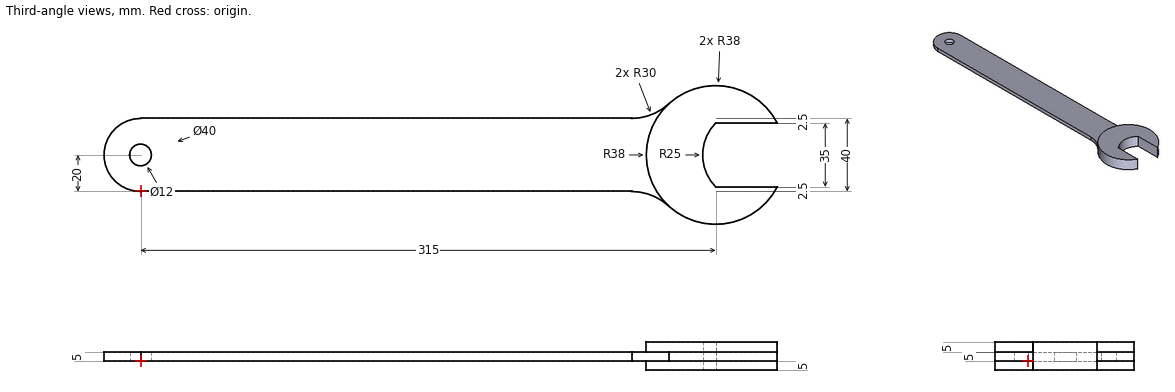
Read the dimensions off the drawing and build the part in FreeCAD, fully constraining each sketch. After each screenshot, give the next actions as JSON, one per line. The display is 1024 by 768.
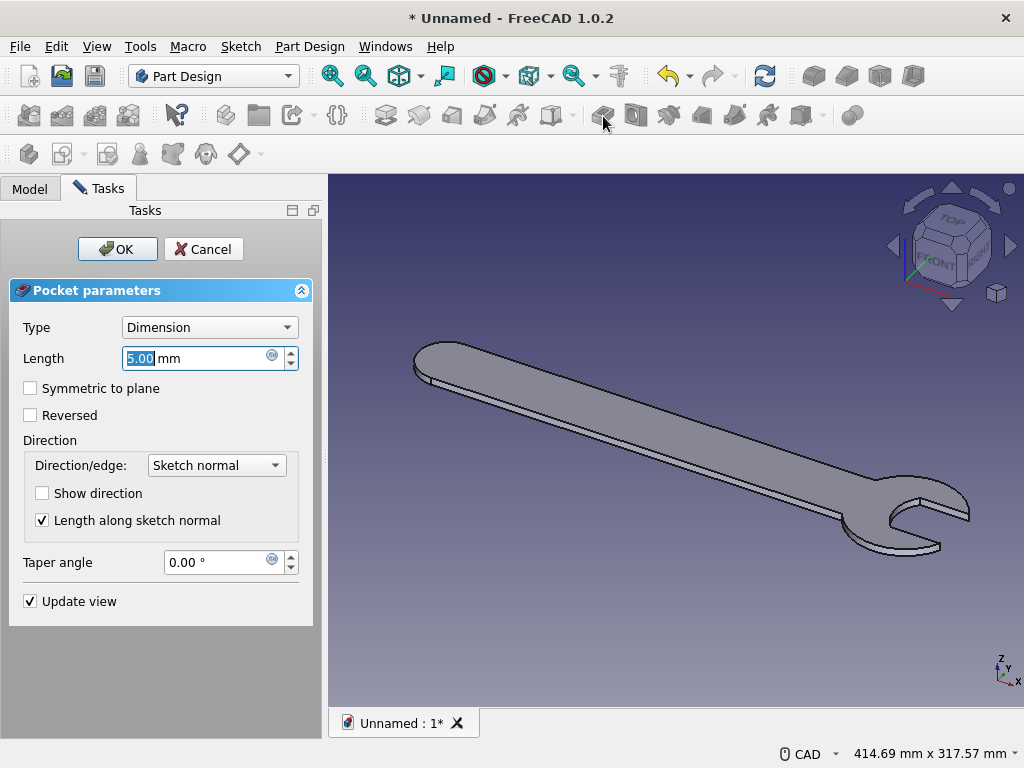
{"action": "type", "text": "5"}
{"action": "key", "text": "Tab"}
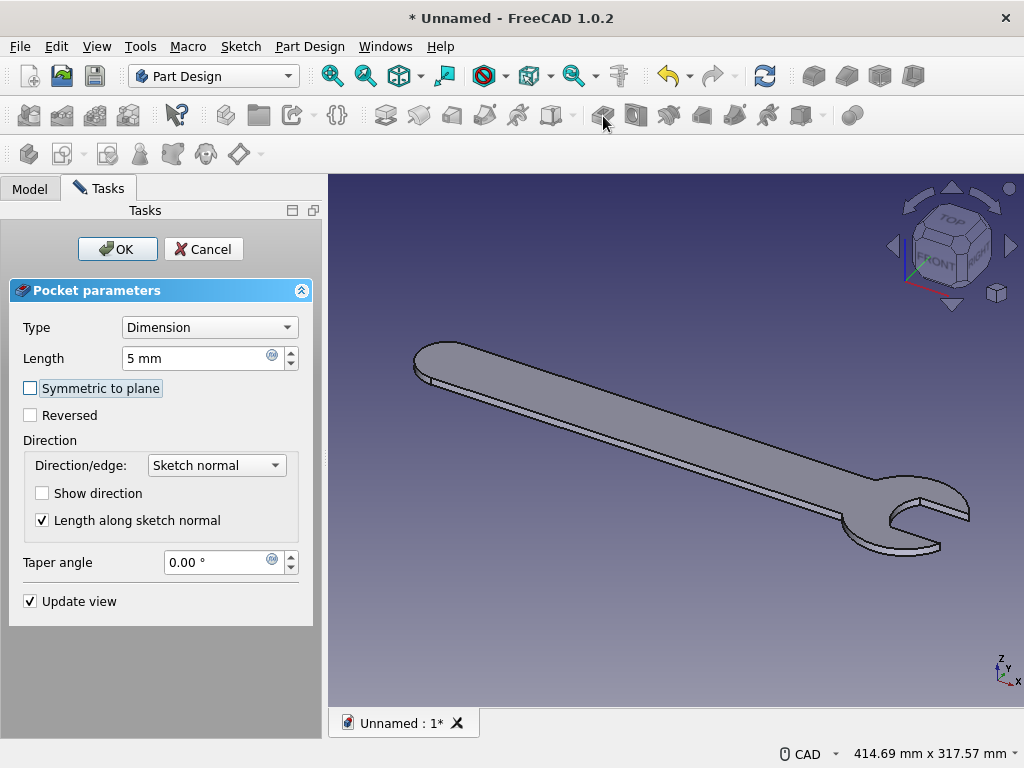
{"action": "left_click", "coordinate": [118, 249]}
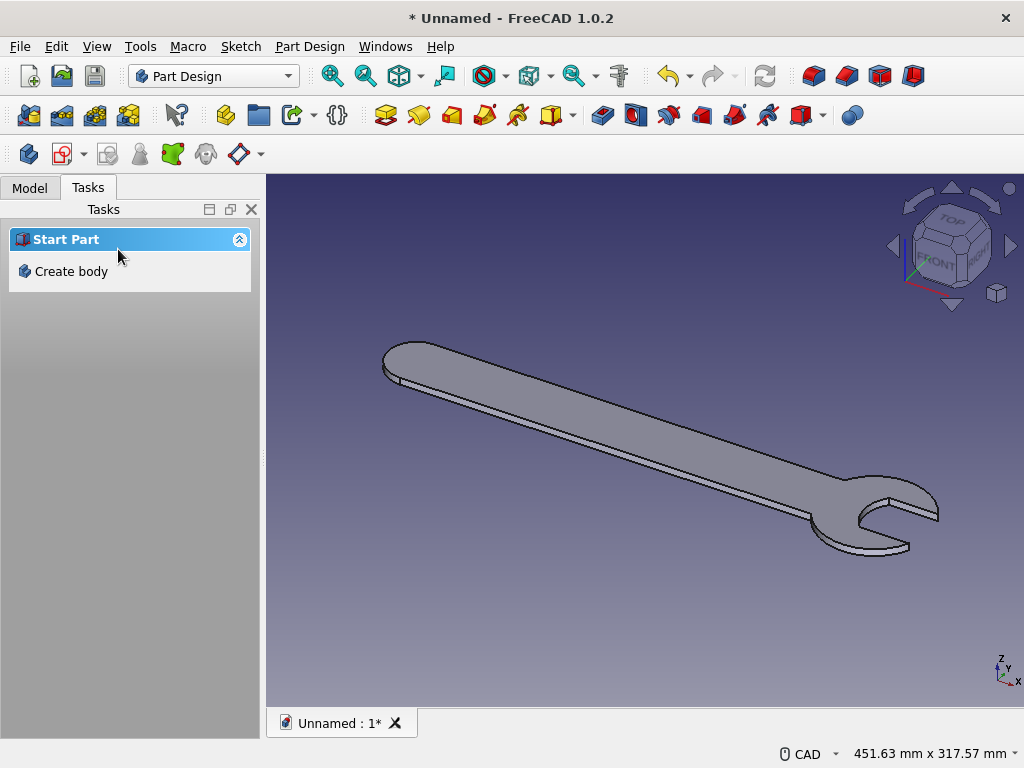
{"action": "left_click", "coordinate": [30, 188]}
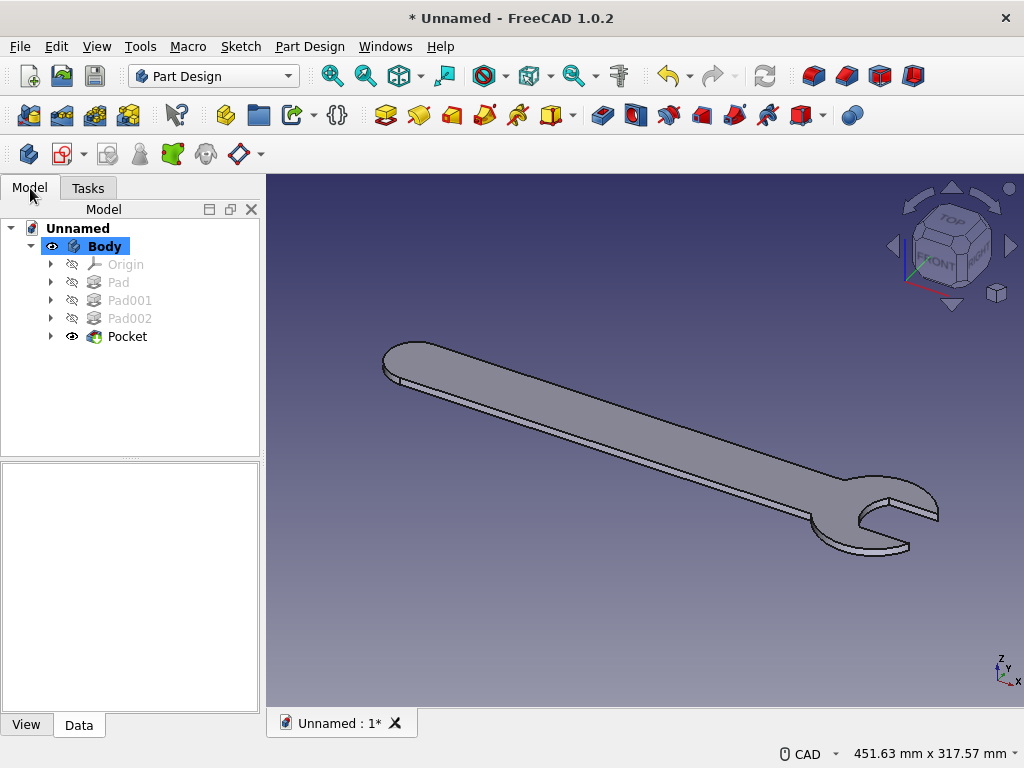
{"action": "left_click", "coordinate": [51, 264]}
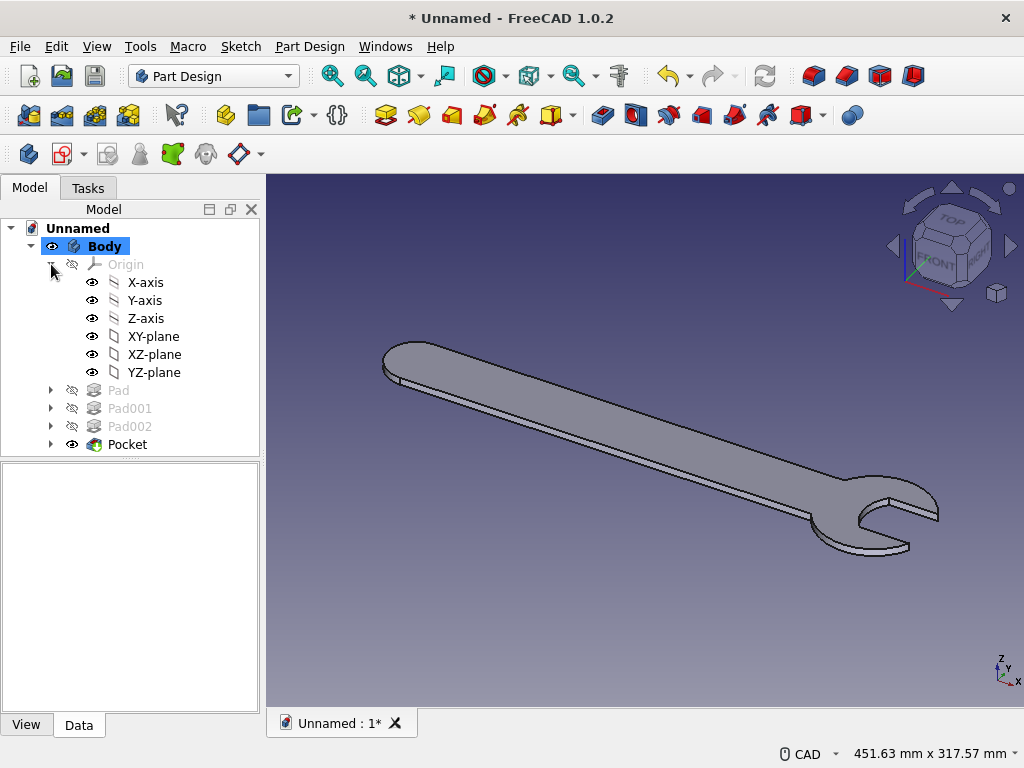
{"action": "left_click", "coordinate": [137, 336]}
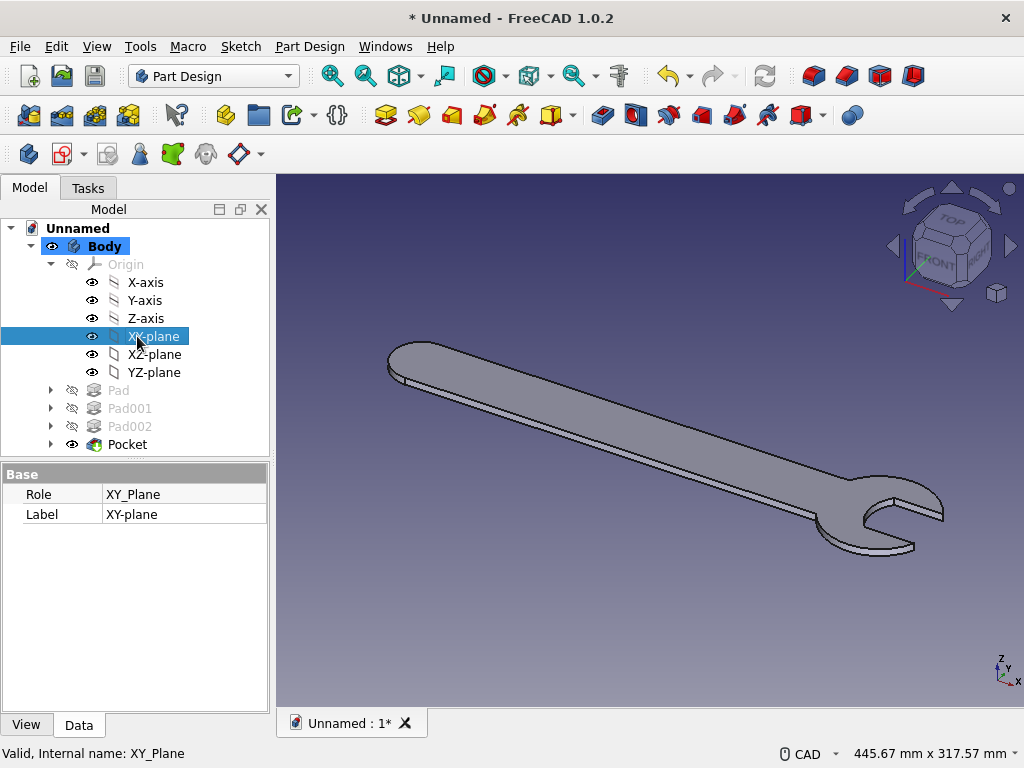
{"action": "left_click", "coordinate": [238, 154]}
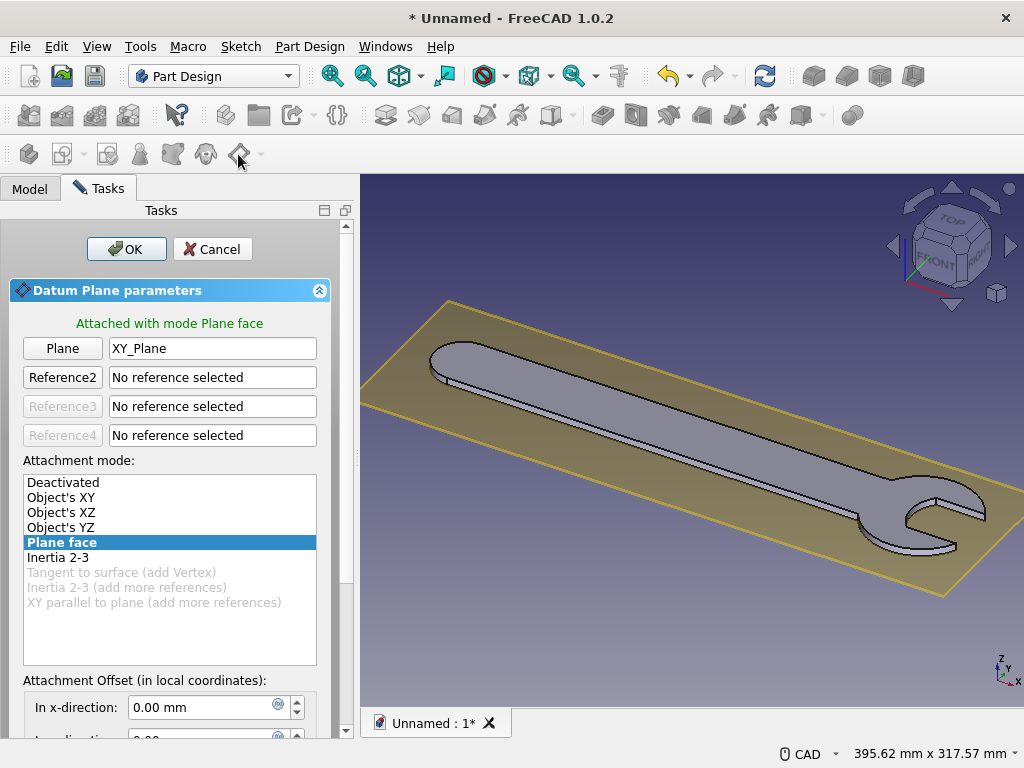
{"action": "scroll", "coordinate": [346, 479], "scroll_direction": "down", "scroll_amount": 2}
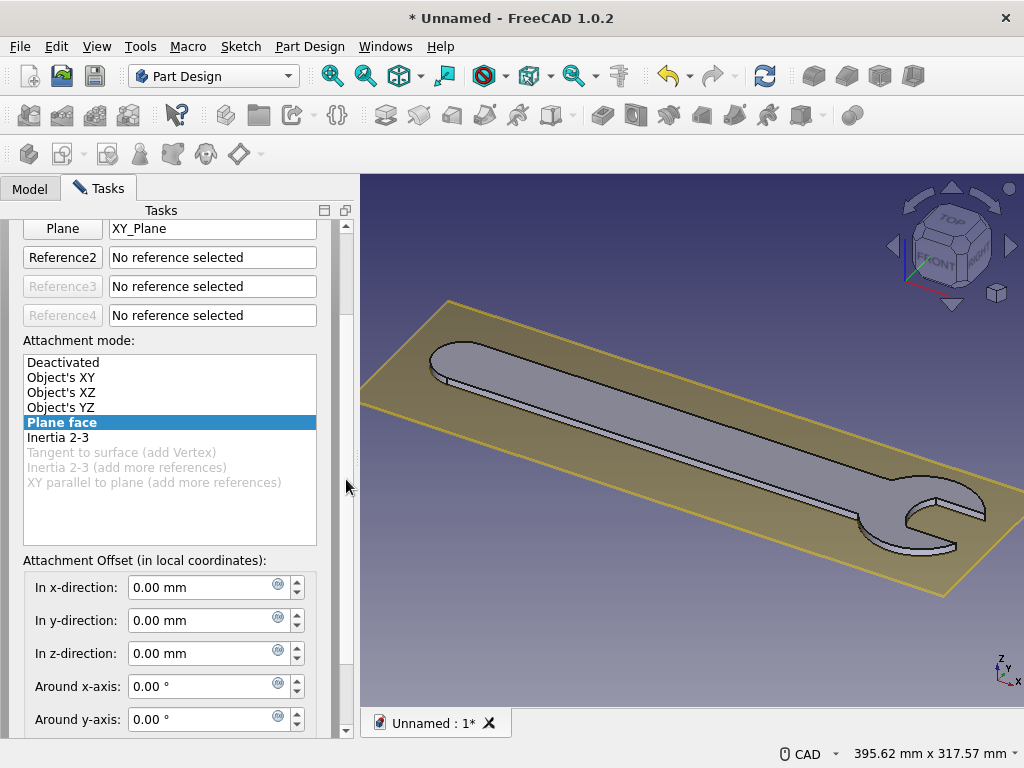
{"action": "triple_click", "coordinate": [210, 654]}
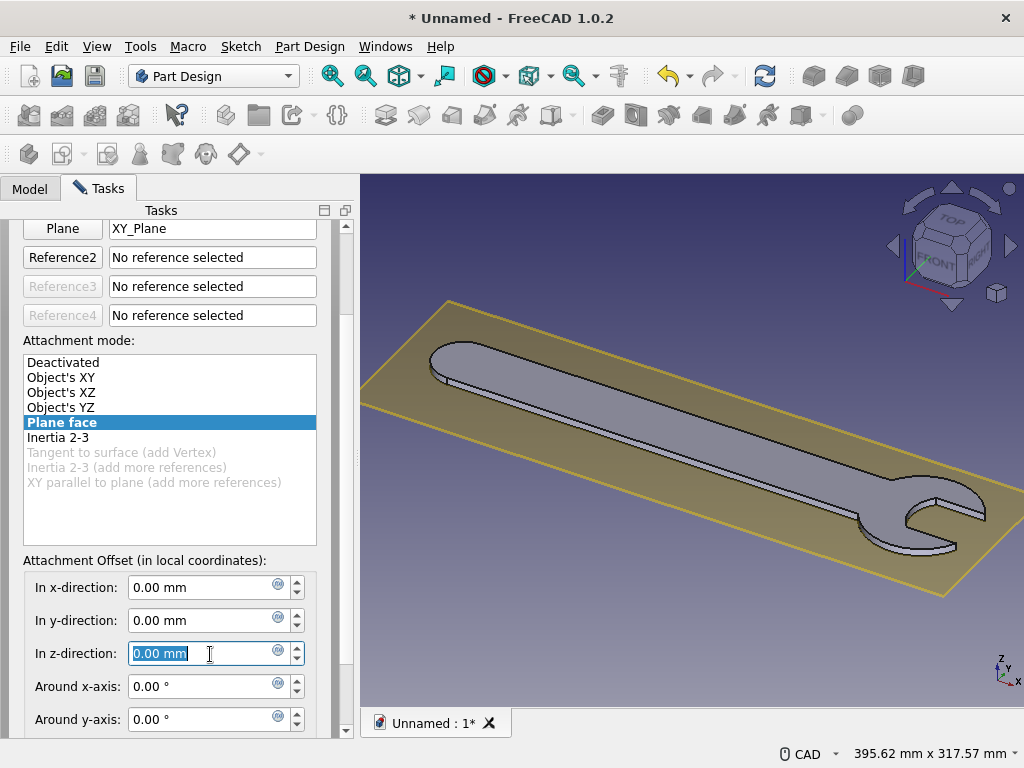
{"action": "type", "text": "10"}
{"action": "key", "text": "Tab"}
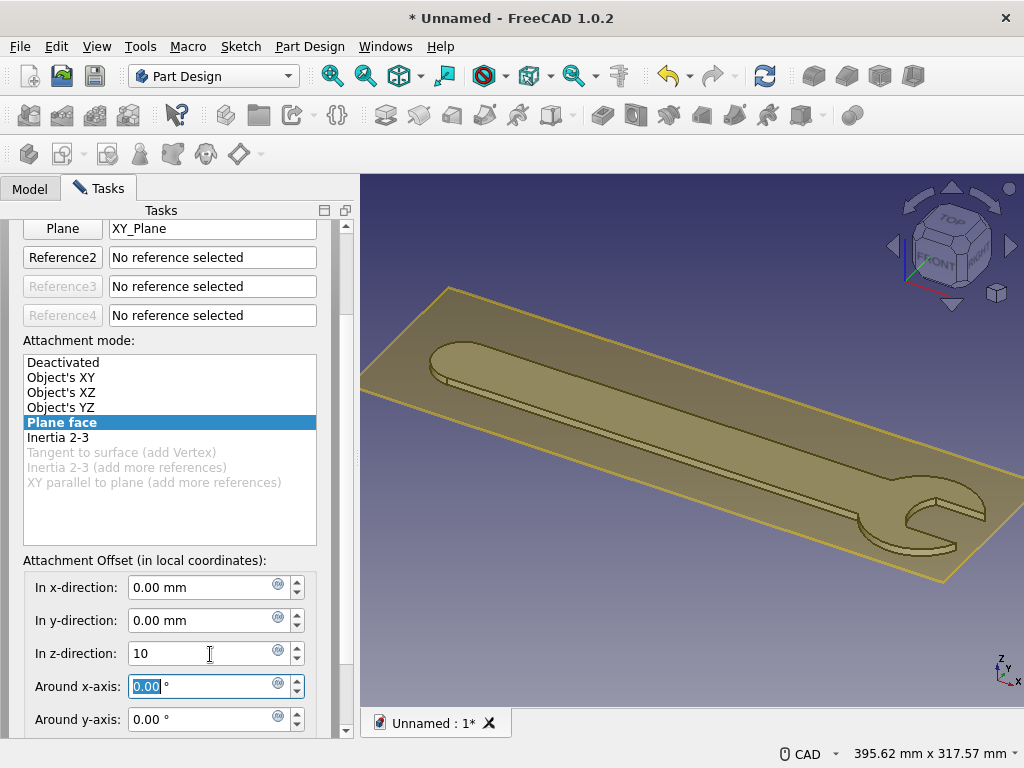
{"action": "scroll", "coordinate": [346, 479], "scroll_direction": "up", "scroll_amount": 3}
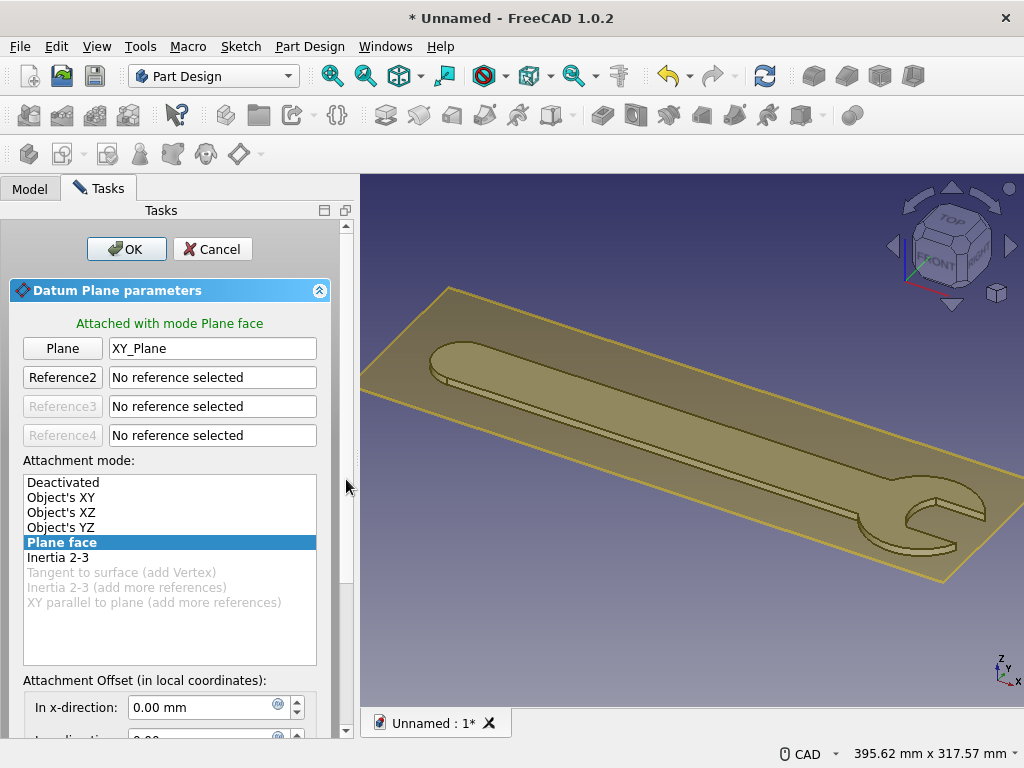
{"action": "left_click", "coordinate": [127, 249]}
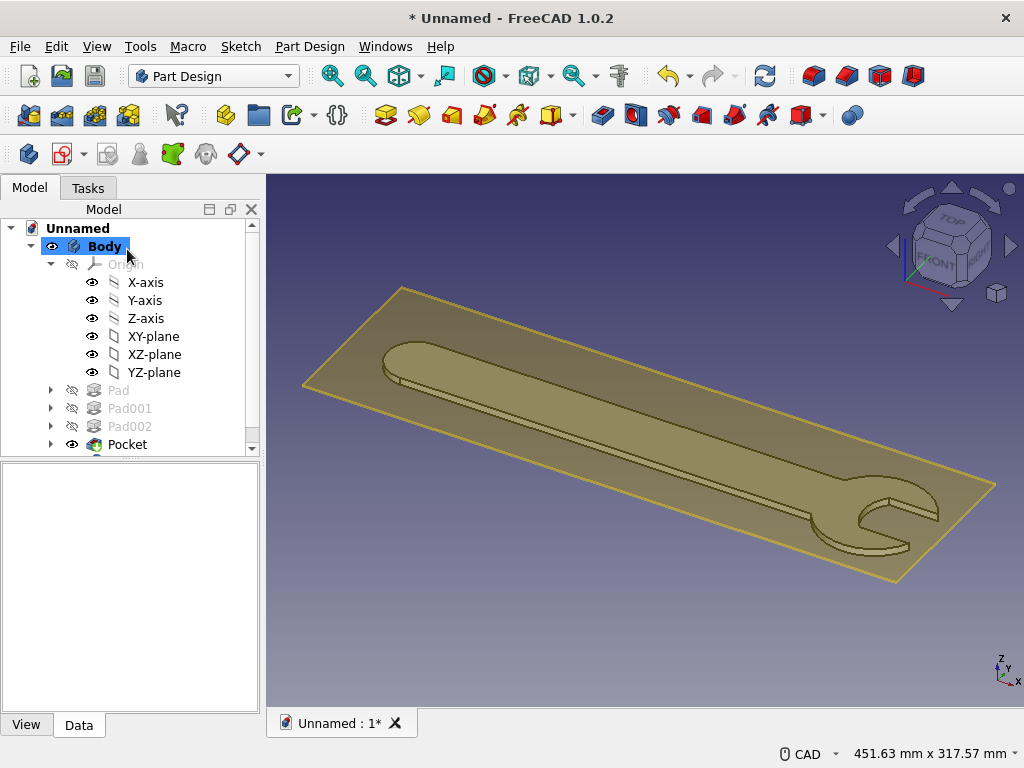
{"action": "scroll", "coordinate": [101, 332], "scroll_direction": "down", "scroll_amount": 3}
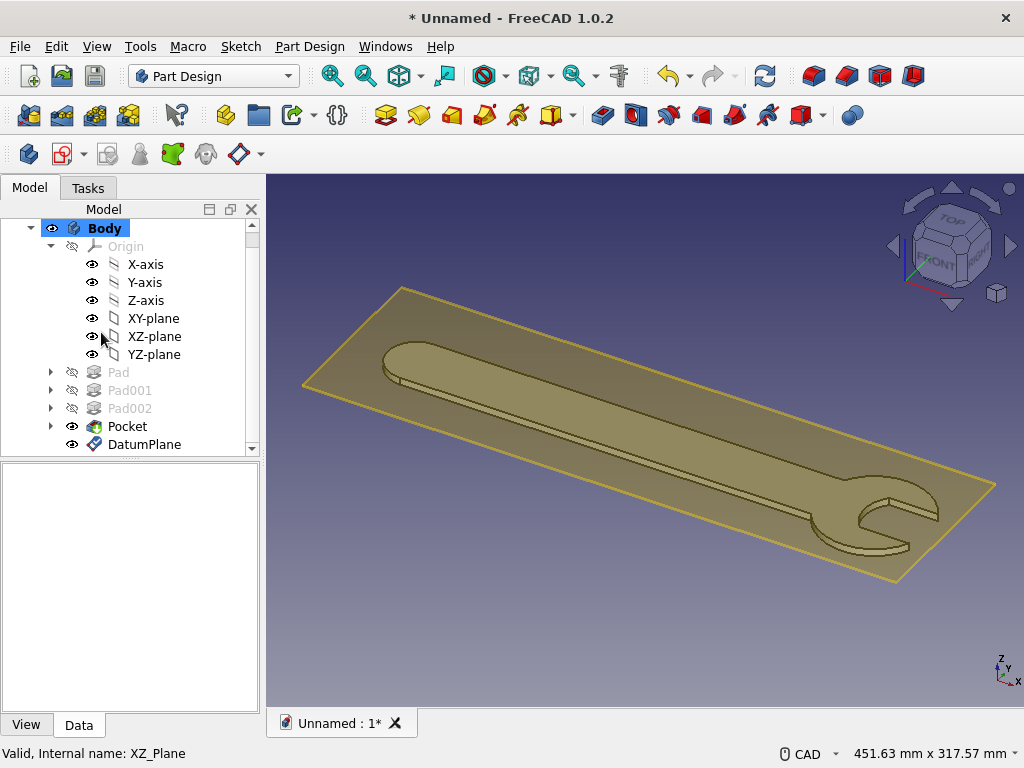
{"action": "left_click", "coordinate": [117, 444]}